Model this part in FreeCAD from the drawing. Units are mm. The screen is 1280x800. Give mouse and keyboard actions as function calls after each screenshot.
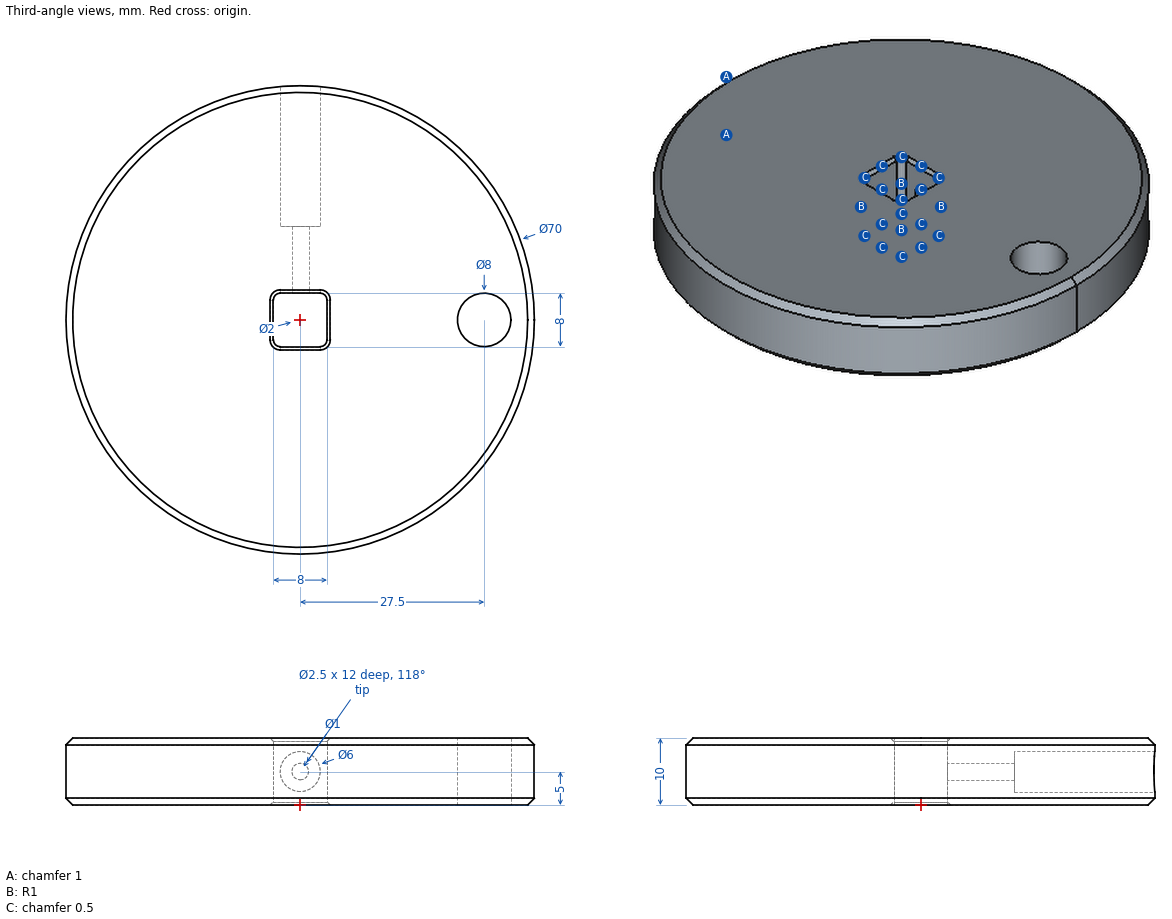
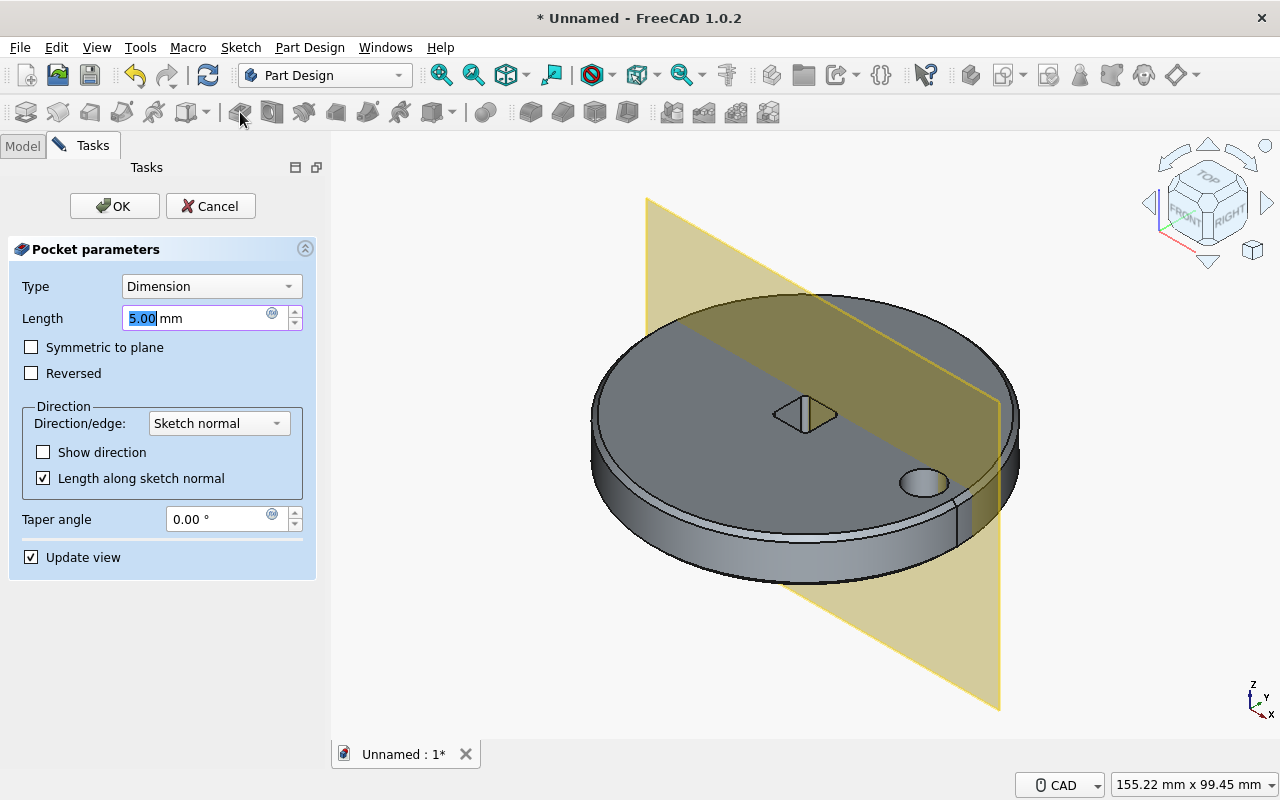
click(212, 286)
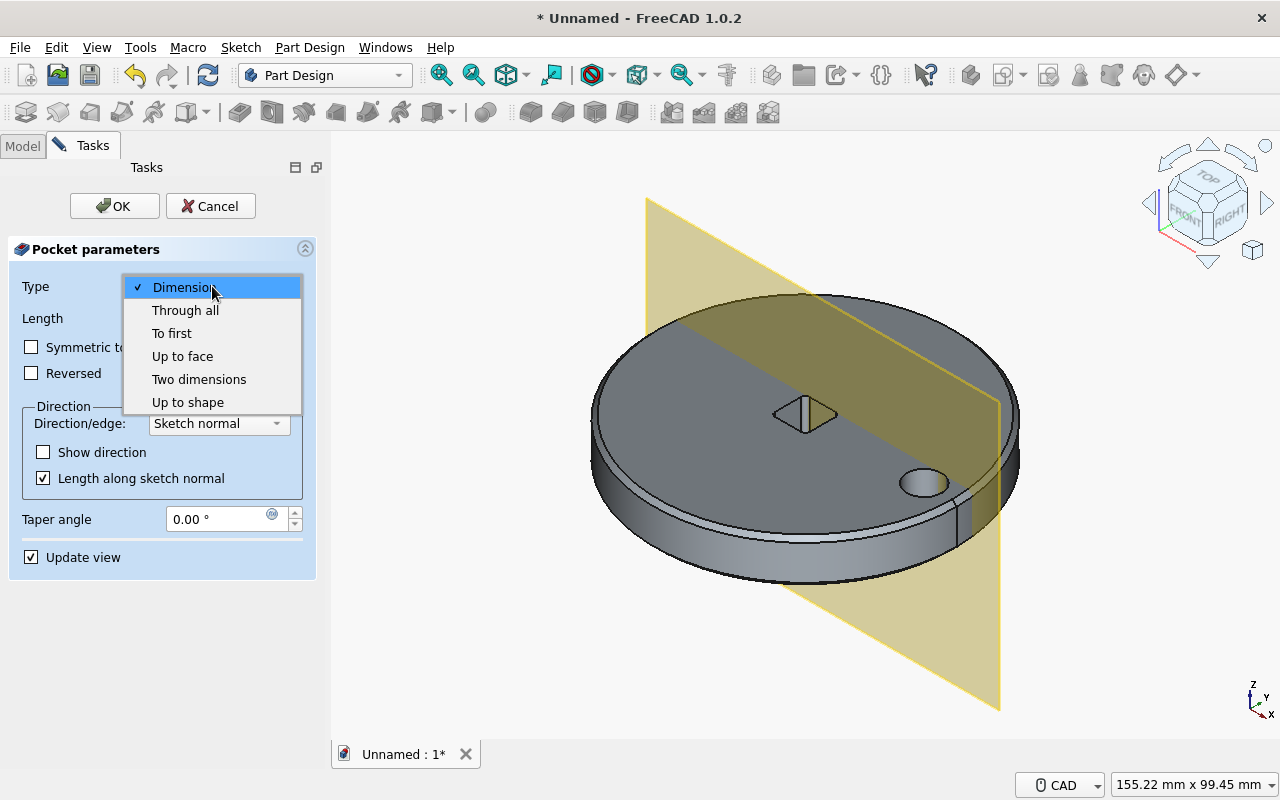
click(212, 310)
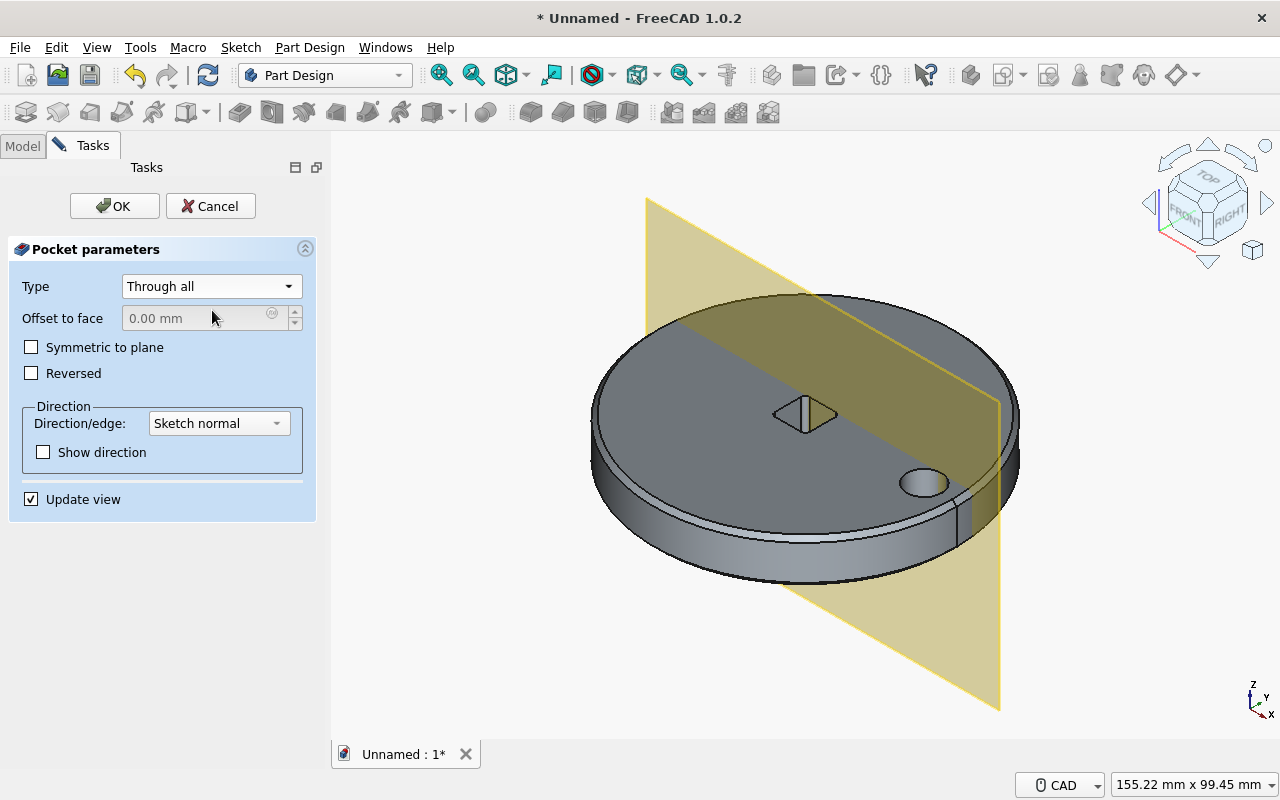
click(115, 206)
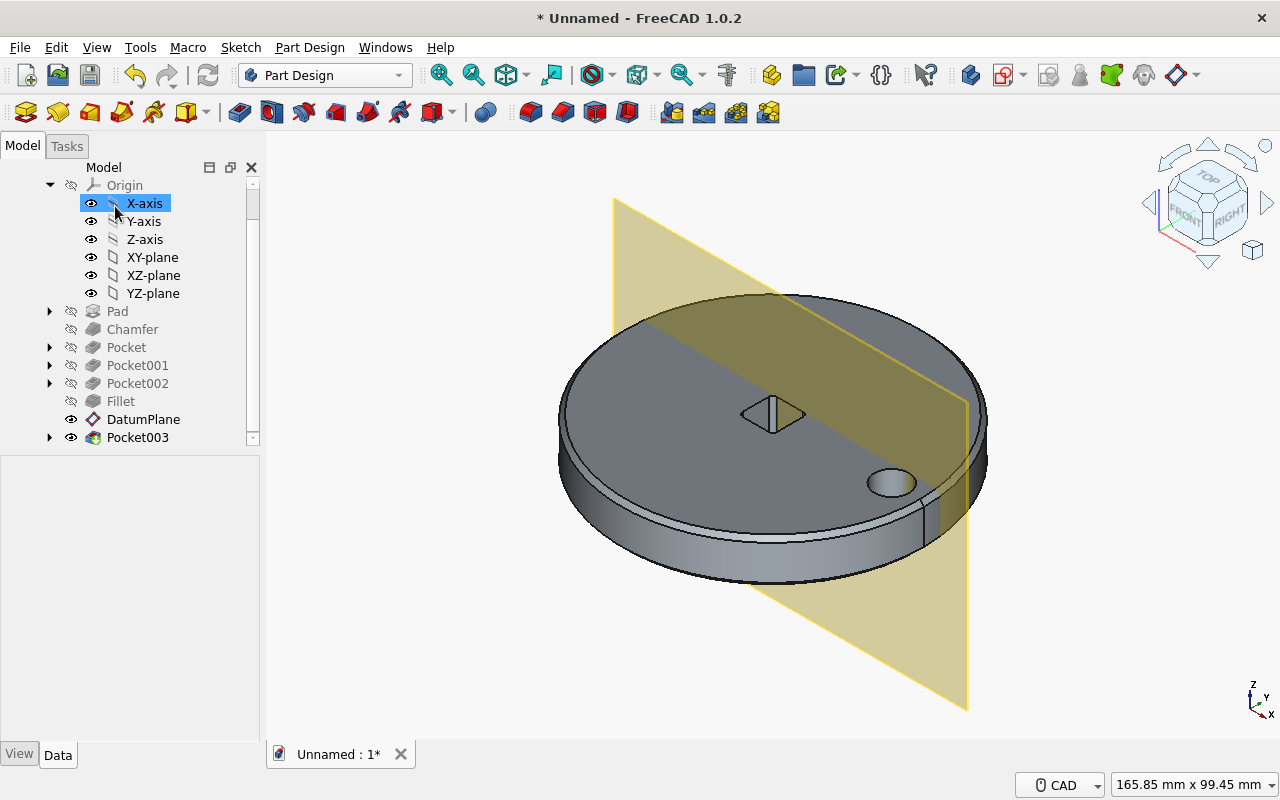
click(116, 419)
key(space)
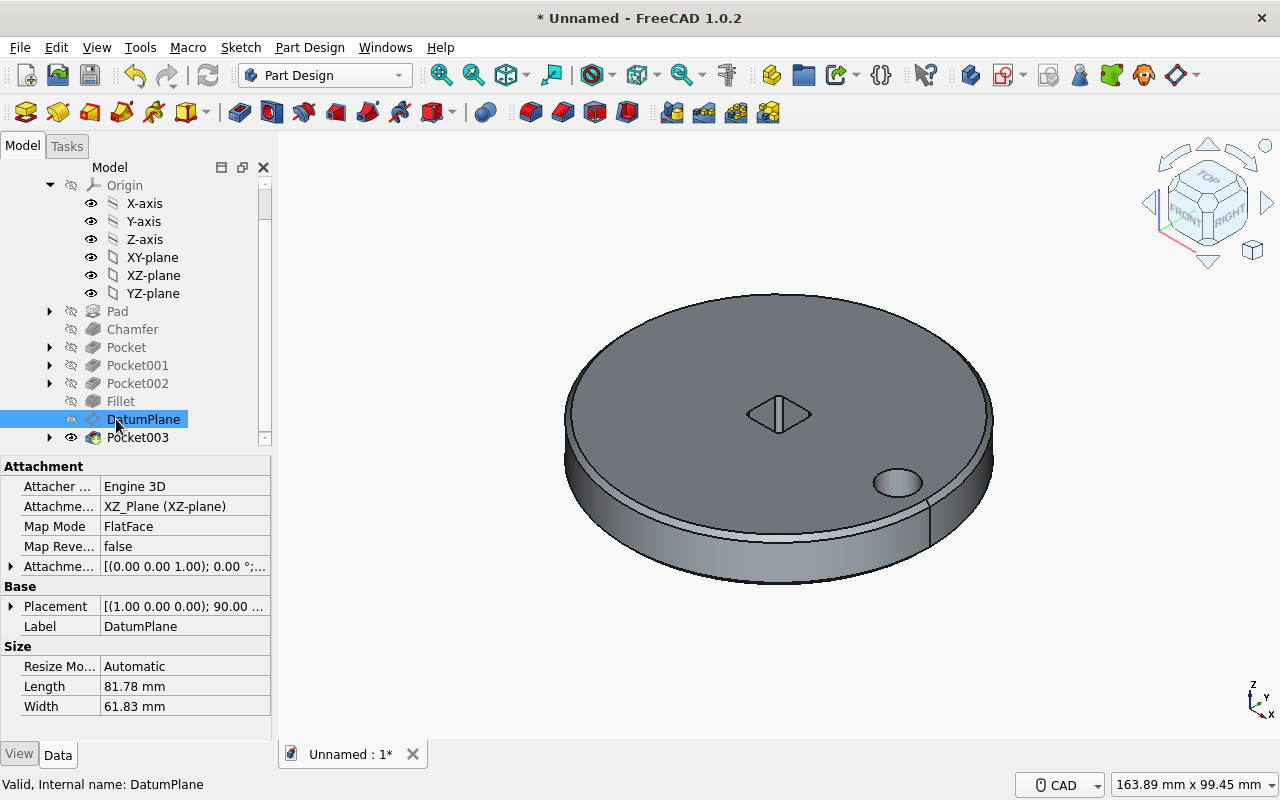
click(136, 275)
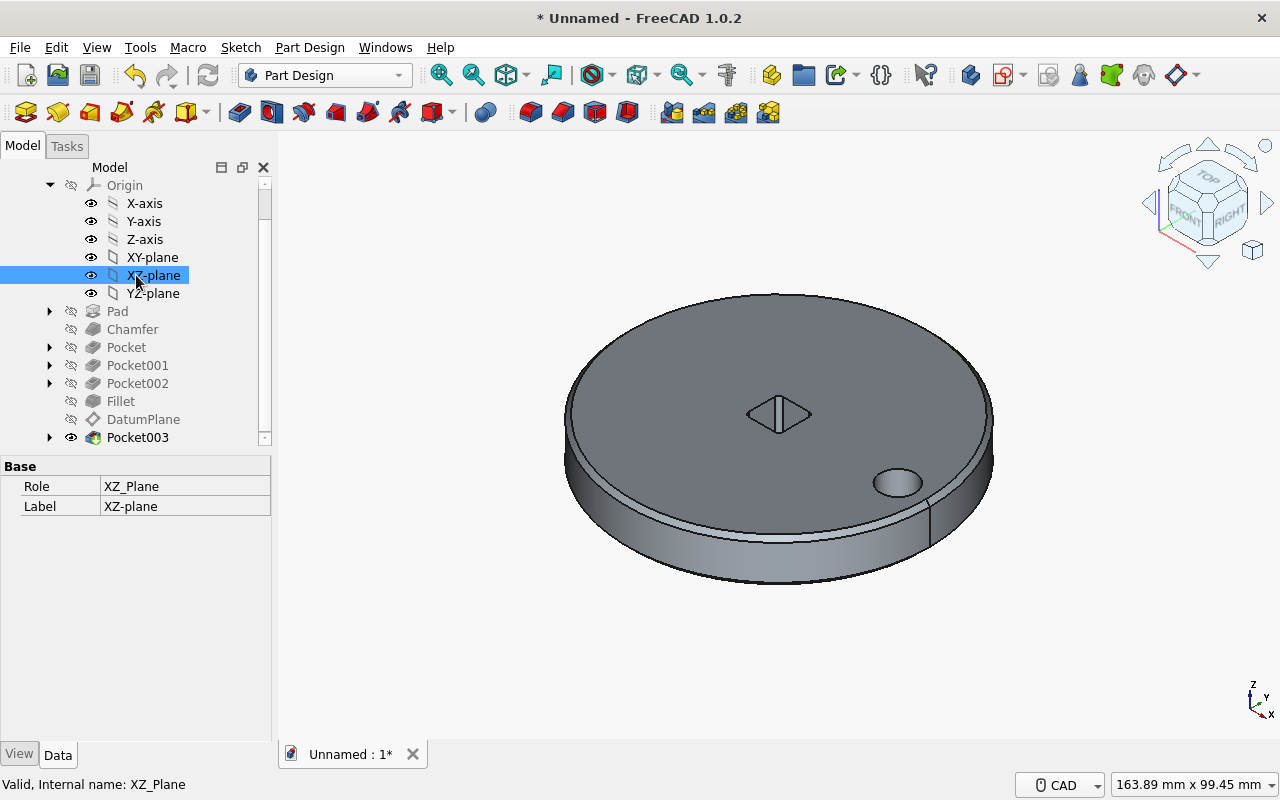
click(1176, 76)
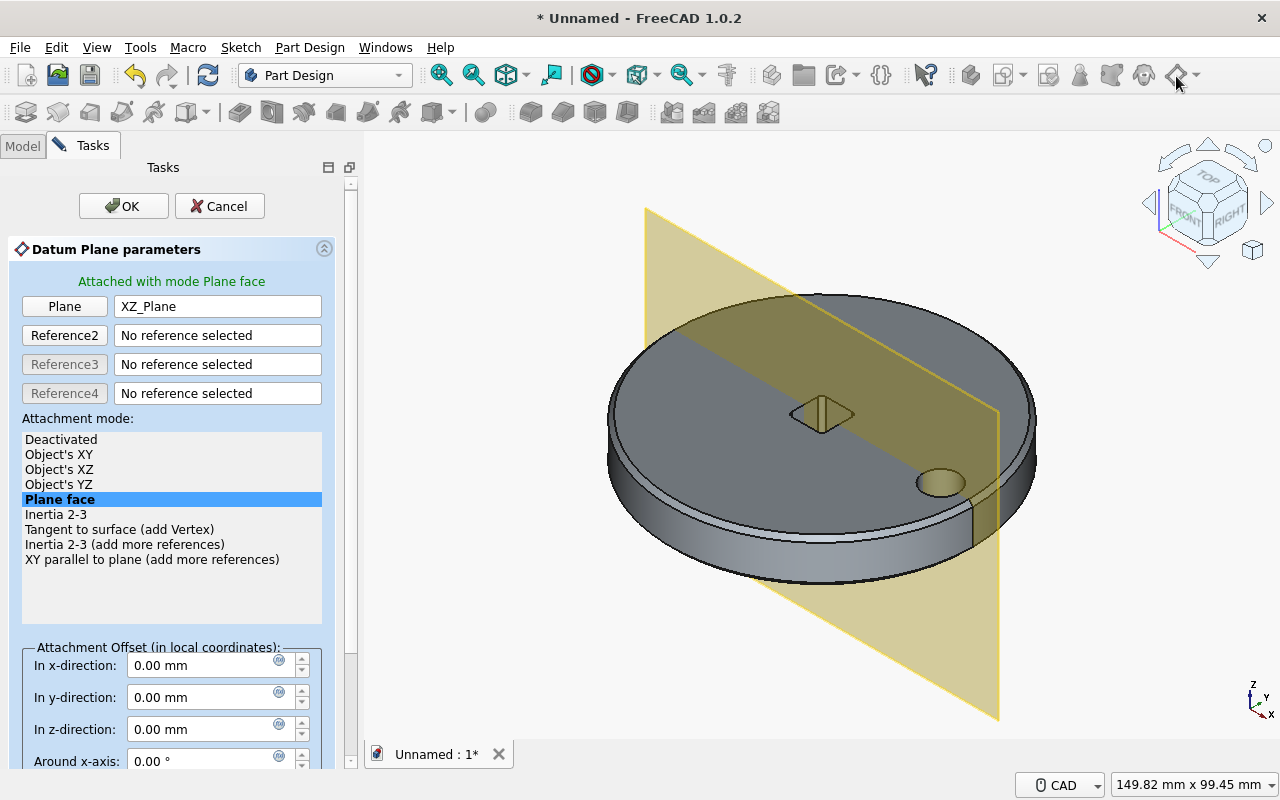
triple_click(210, 729)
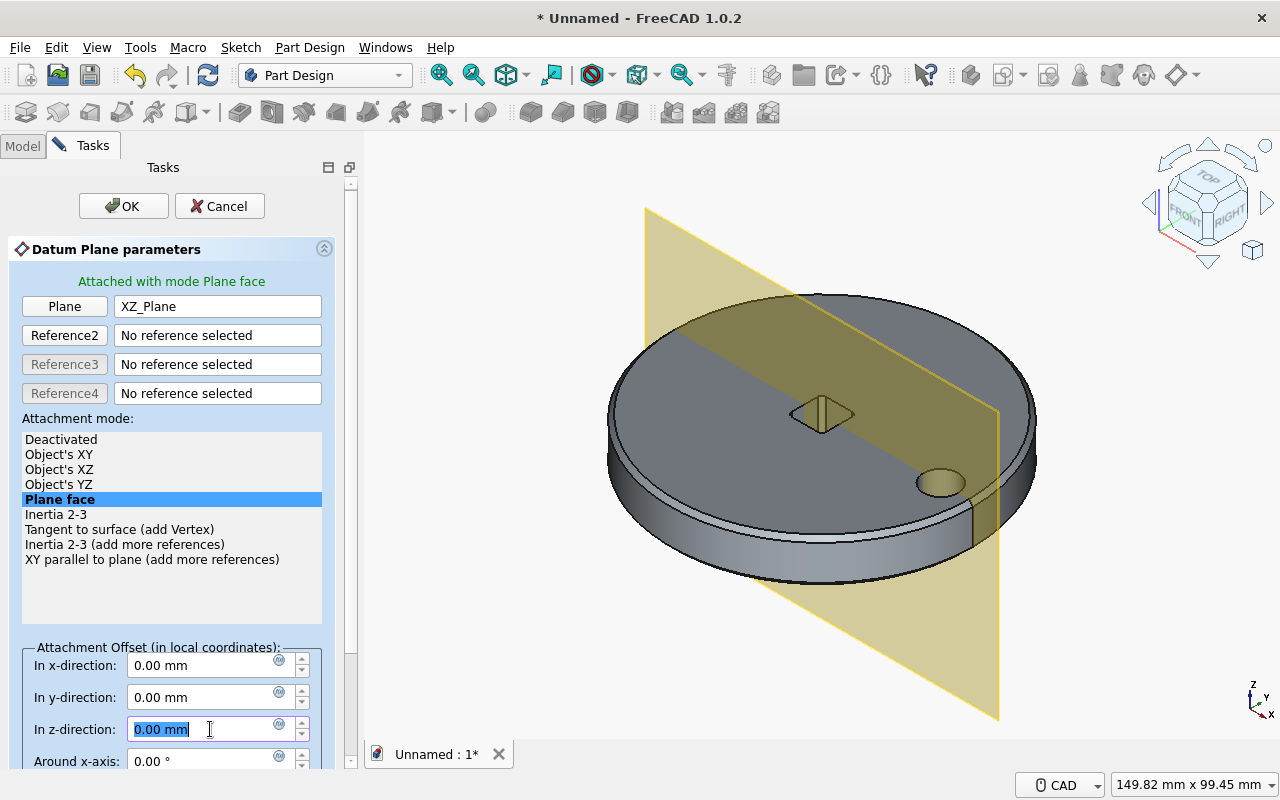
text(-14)
key(Tab)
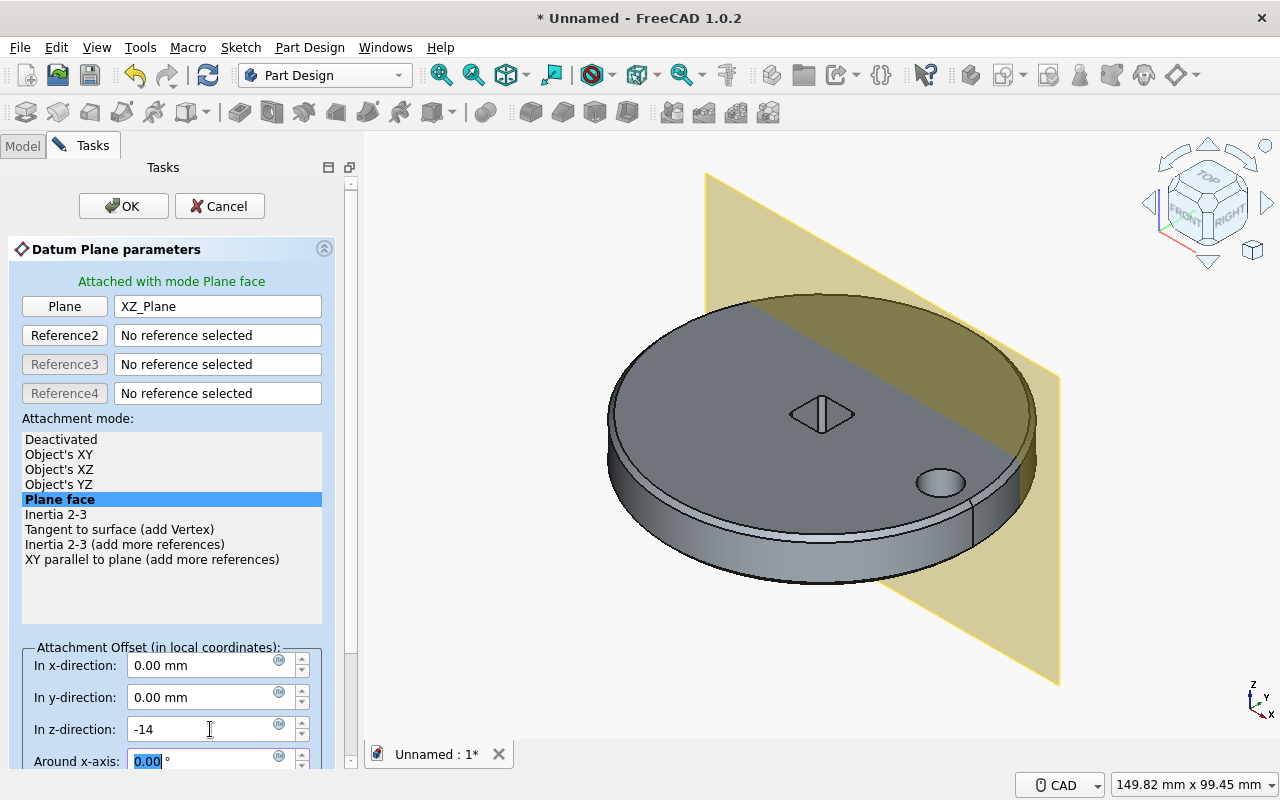
click(124, 206)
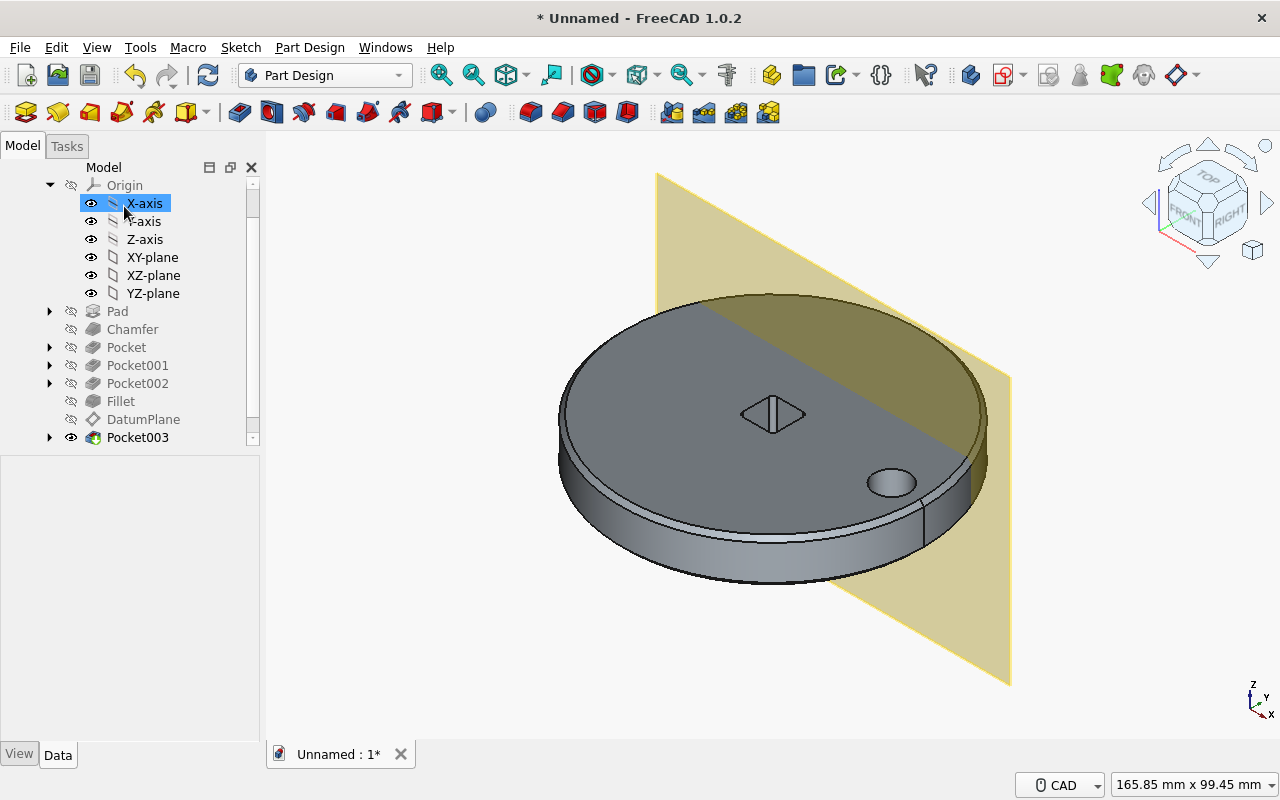
scroll(140, 307, down, 3)